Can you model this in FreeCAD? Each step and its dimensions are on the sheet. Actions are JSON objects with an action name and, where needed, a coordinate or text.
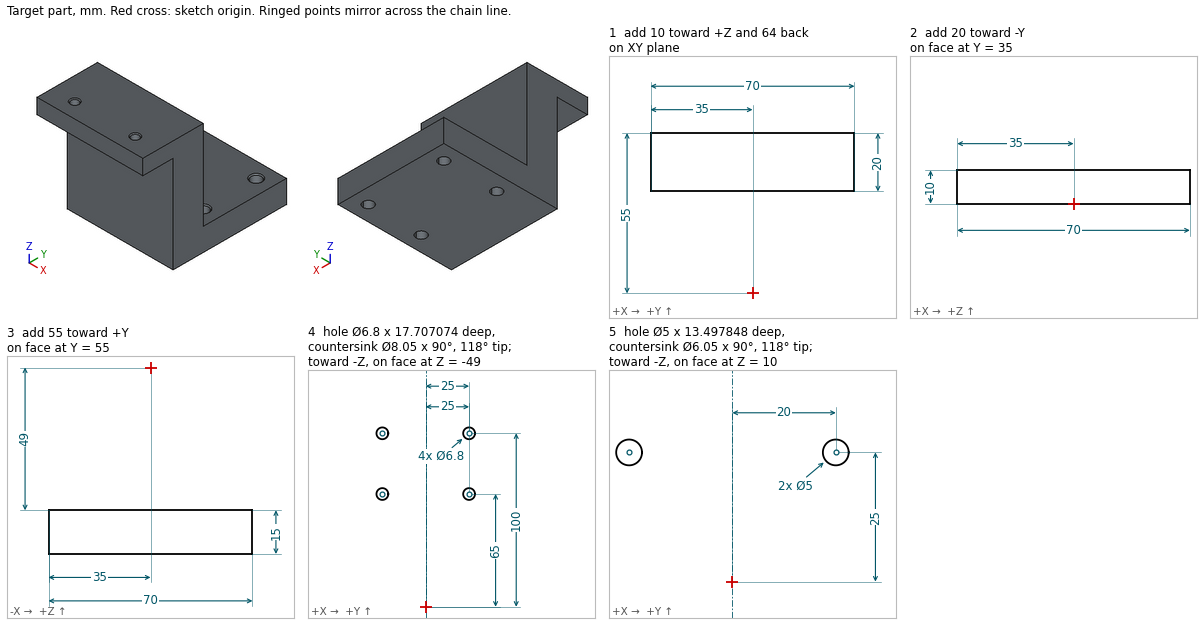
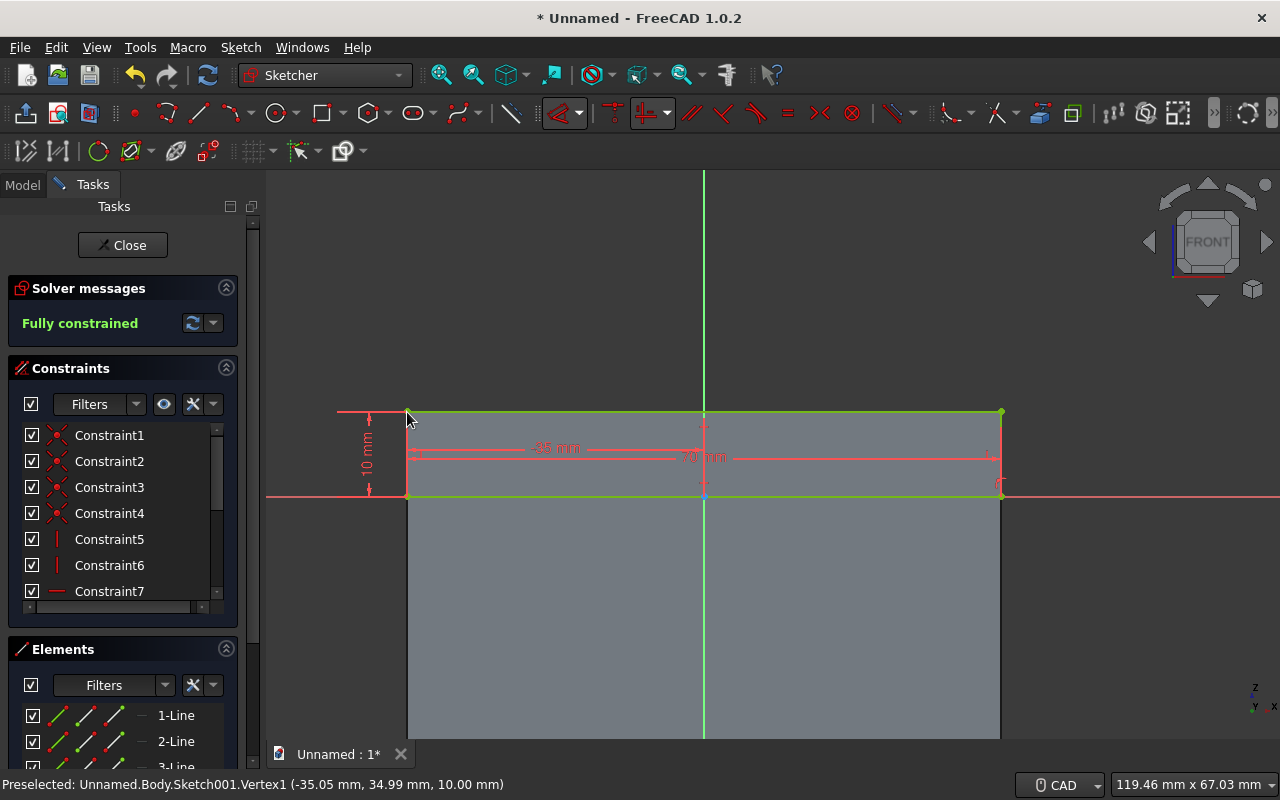
{"action": "left_click", "coordinate": [123, 245]}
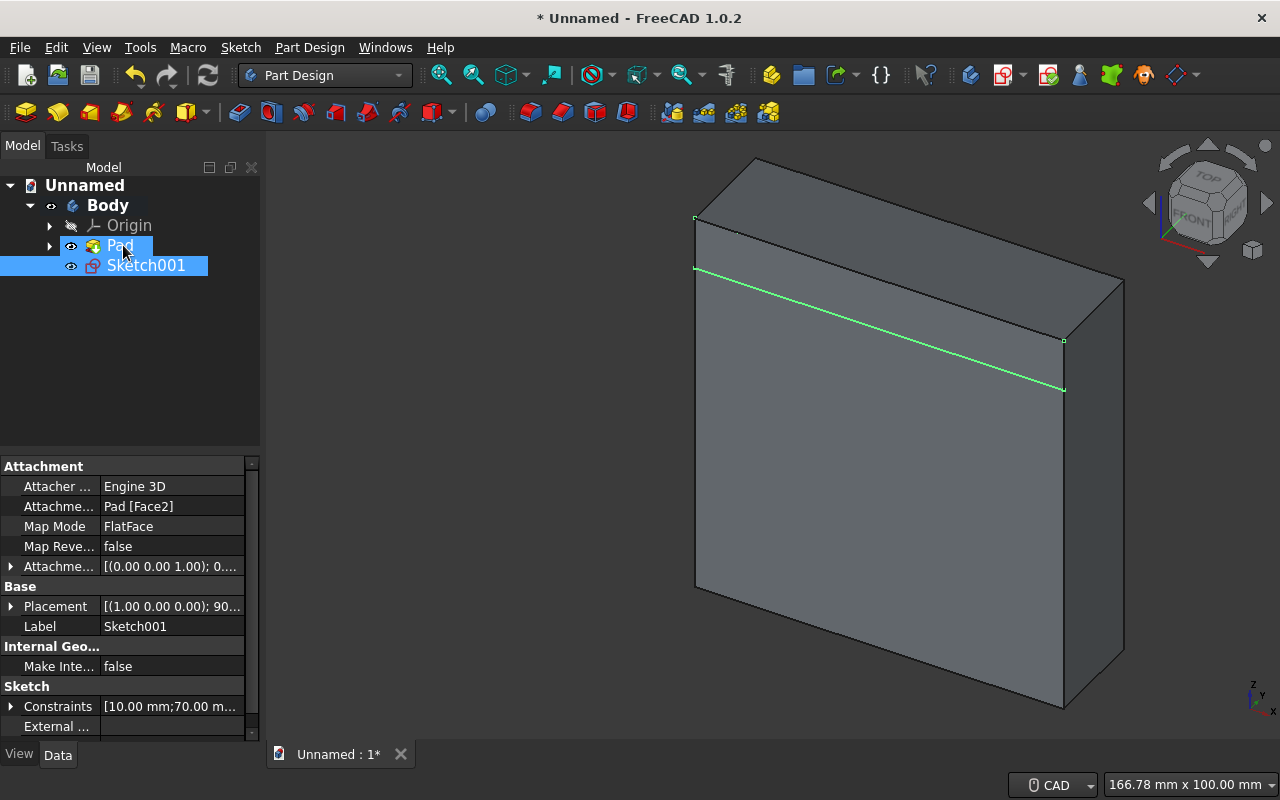
{"action": "left_click", "coordinate": [26, 112]}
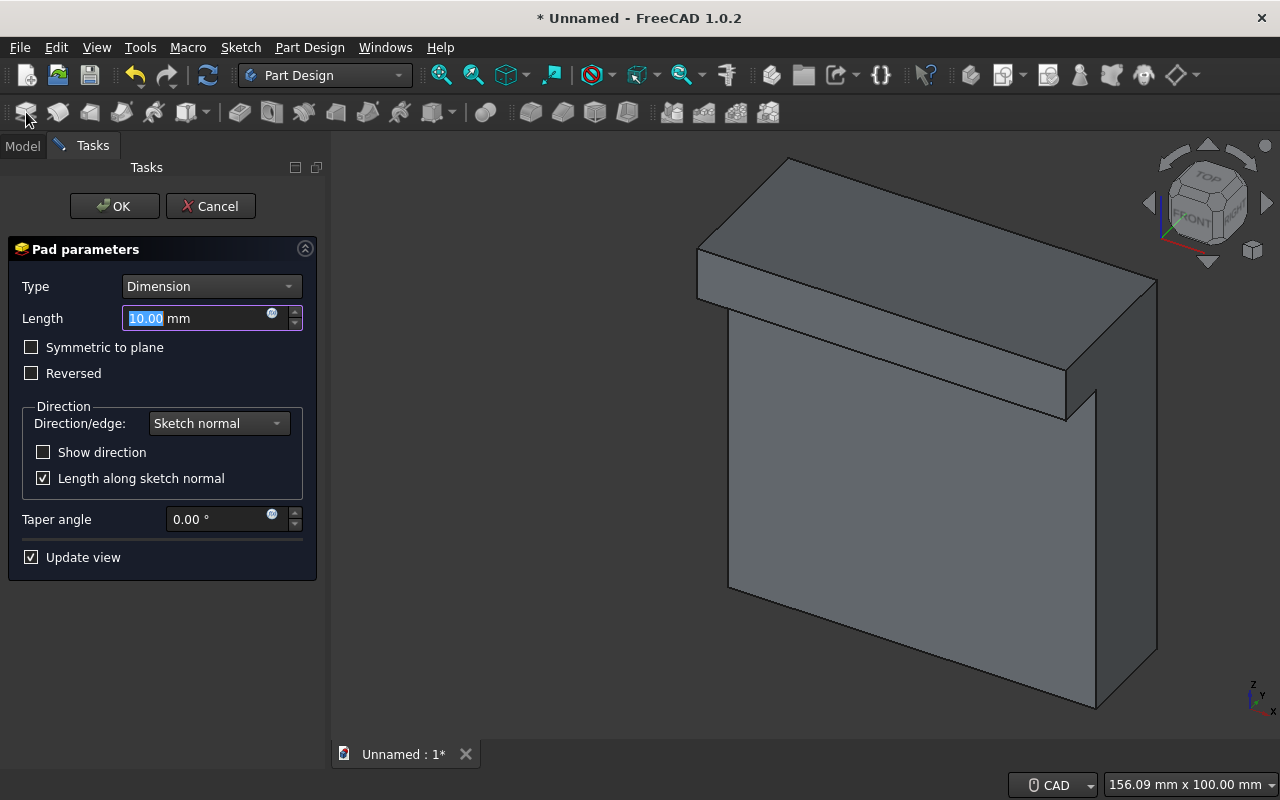
{"action": "type", "text": "20"}
{"action": "key", "text": "Tab"}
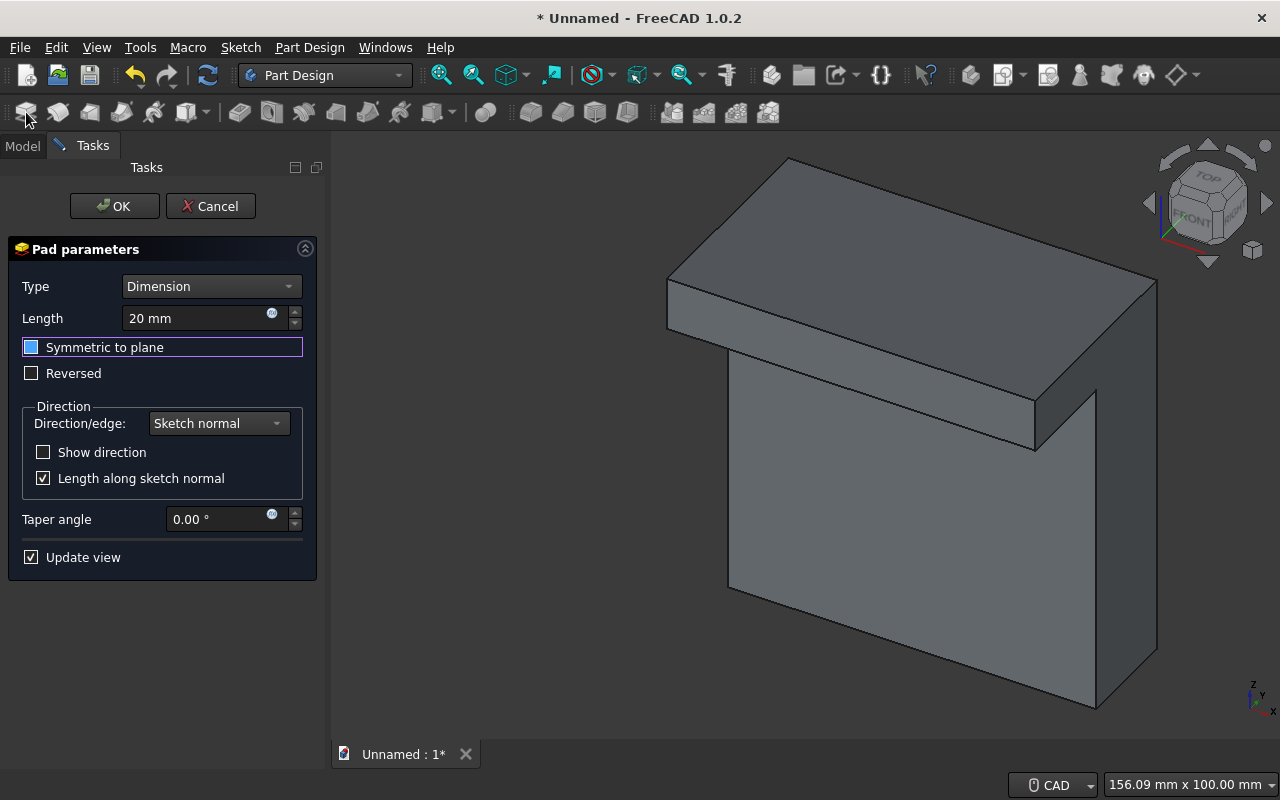
{"action": "left_click", "coordinate": [115, 206]}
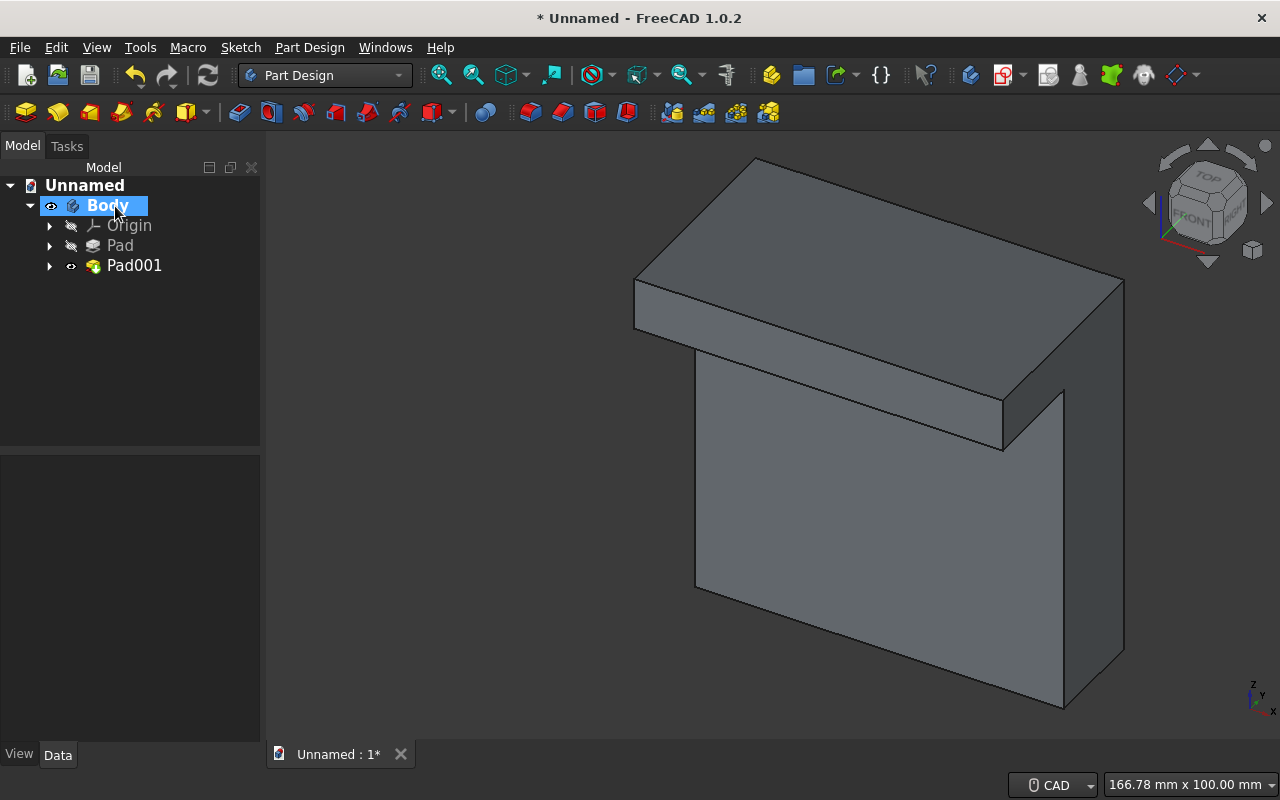
{"action": "key", "text": "v f"}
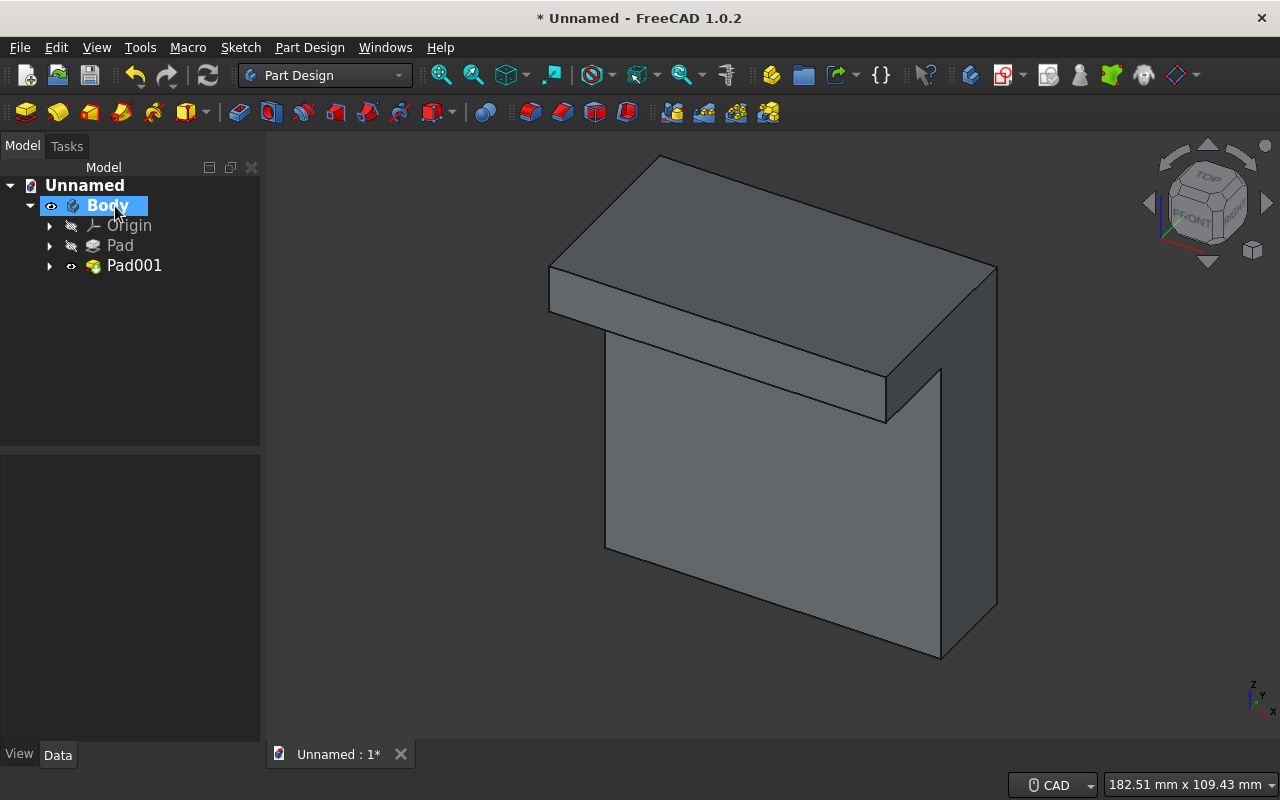
{"action": "key", "text": "4"}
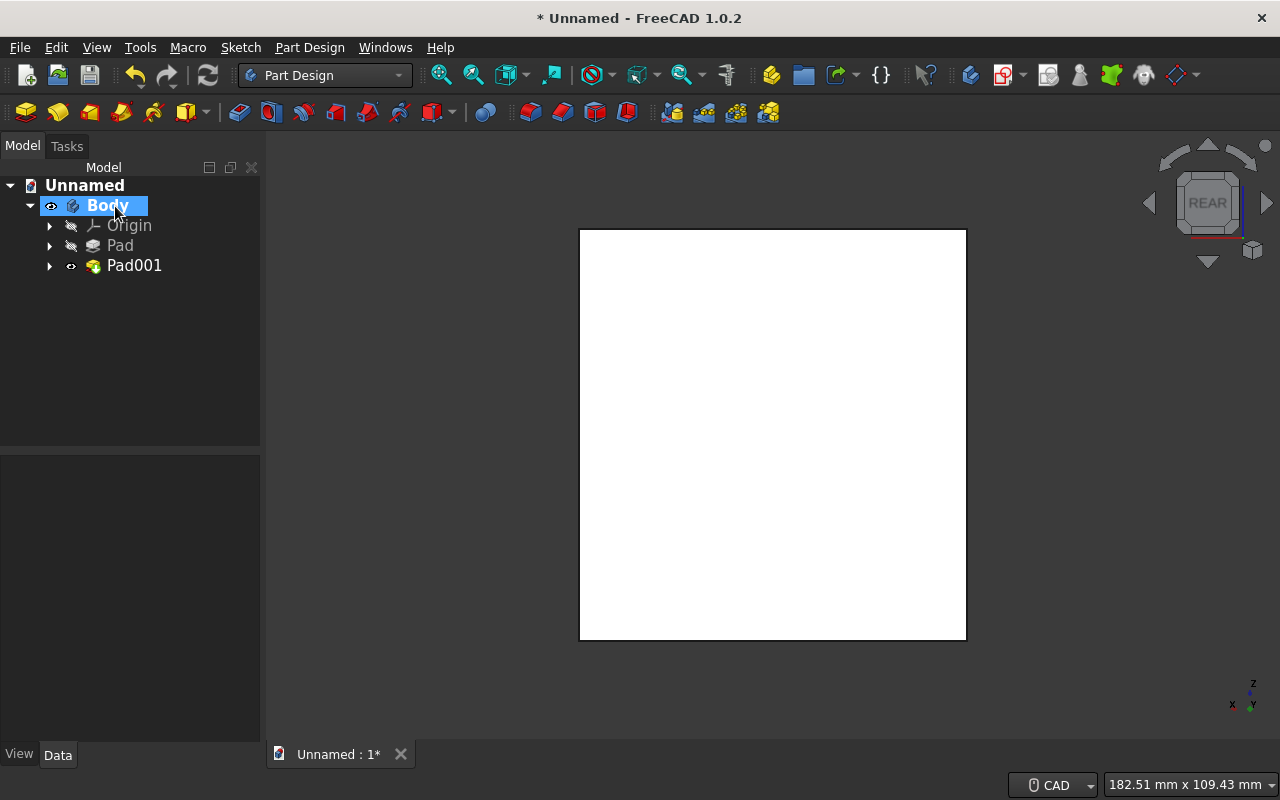
{"action": "left_click", "coordinate": [773, 434]}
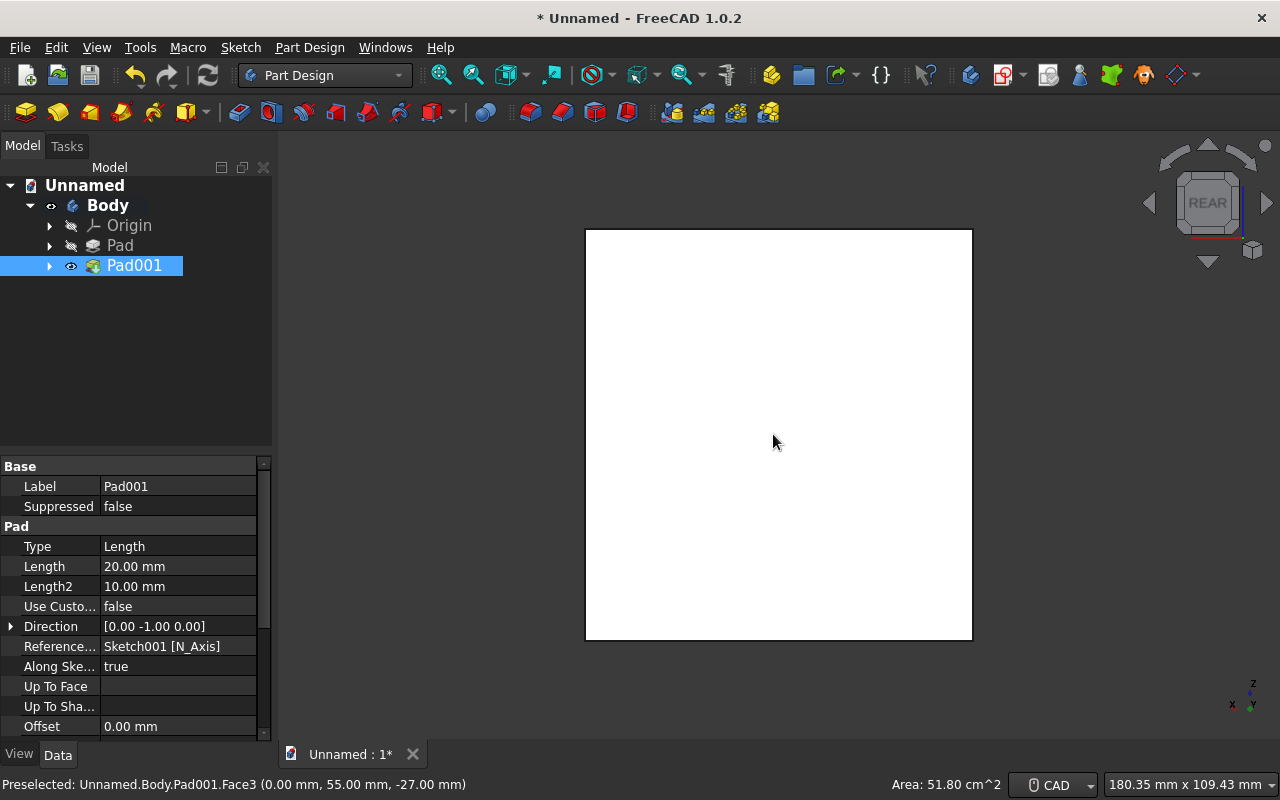
{"action": "left_click", "coordinate": [1004, 76]}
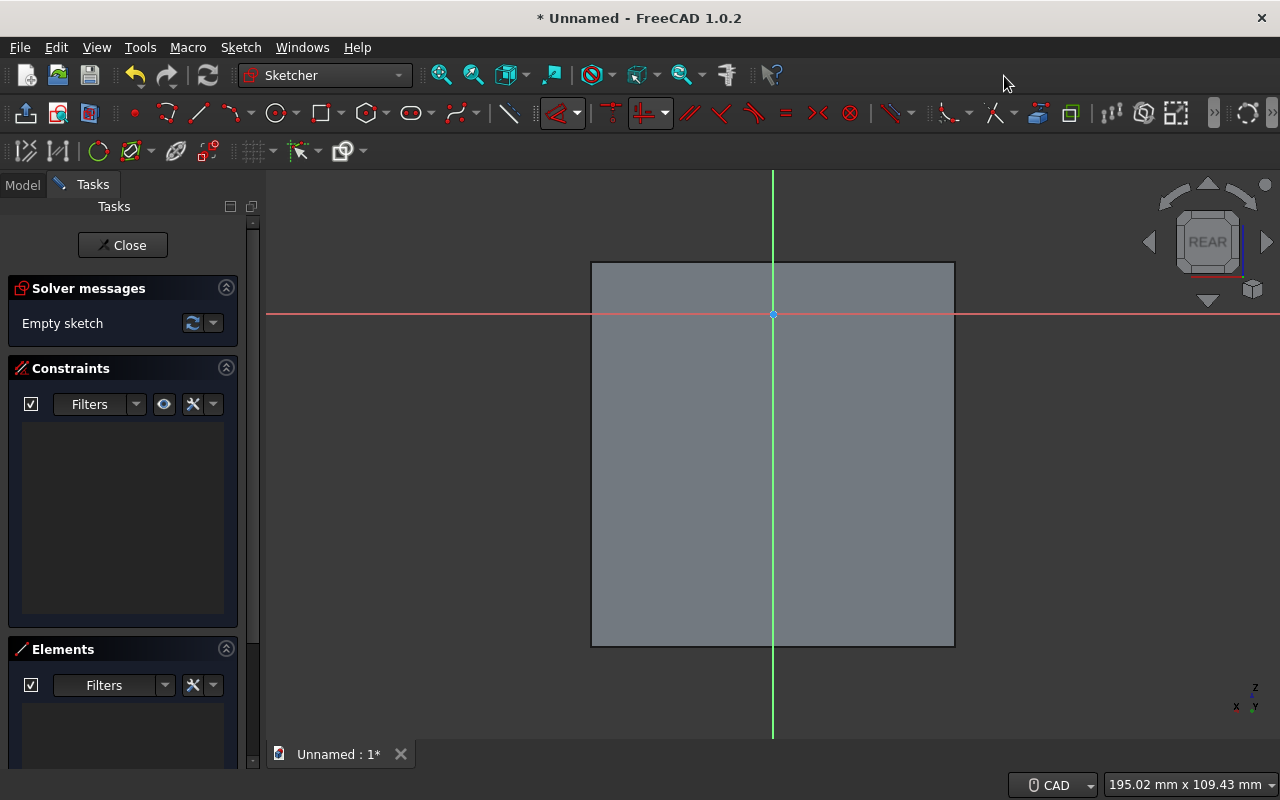
{"action": "left_click", "coordinate": [322, 114]}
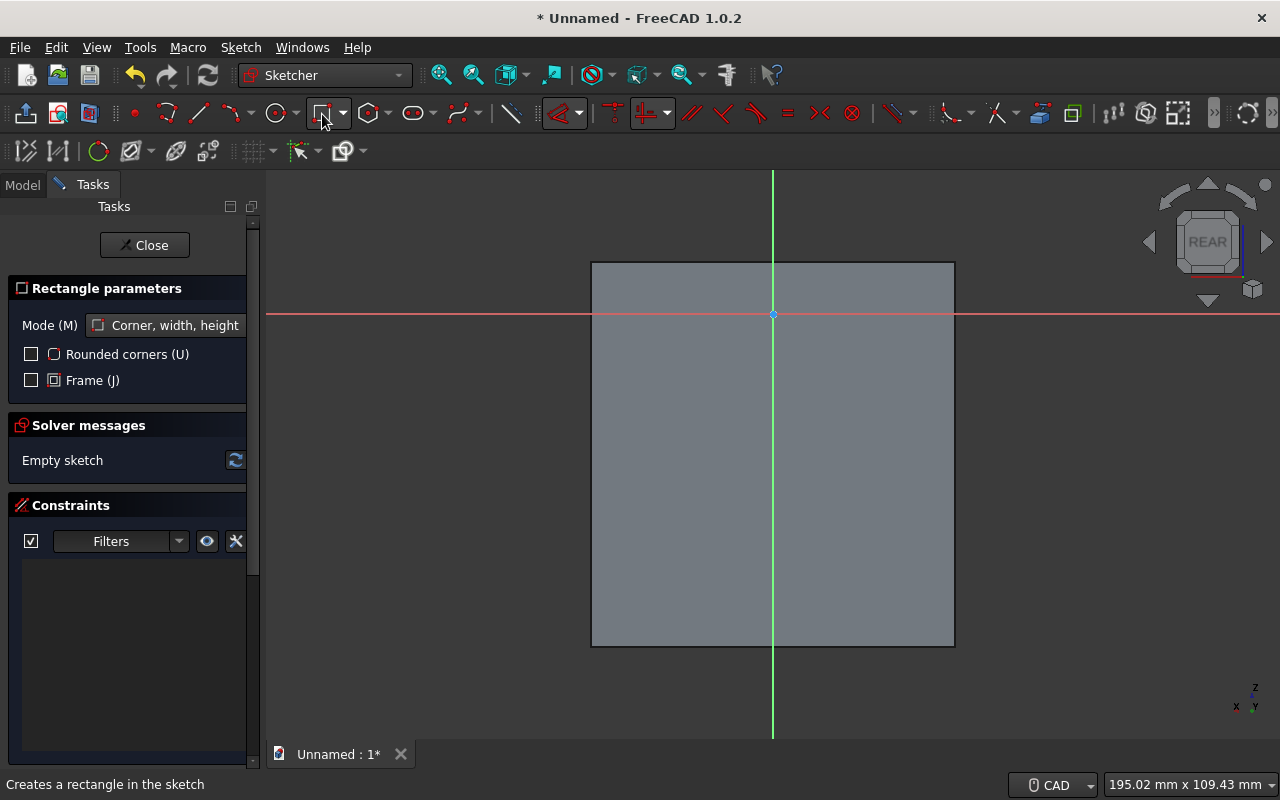
{"action": "left_click", "coordinate": [591, 569]}
{"action": "mouse_move", "coordinate": [955, 647]}